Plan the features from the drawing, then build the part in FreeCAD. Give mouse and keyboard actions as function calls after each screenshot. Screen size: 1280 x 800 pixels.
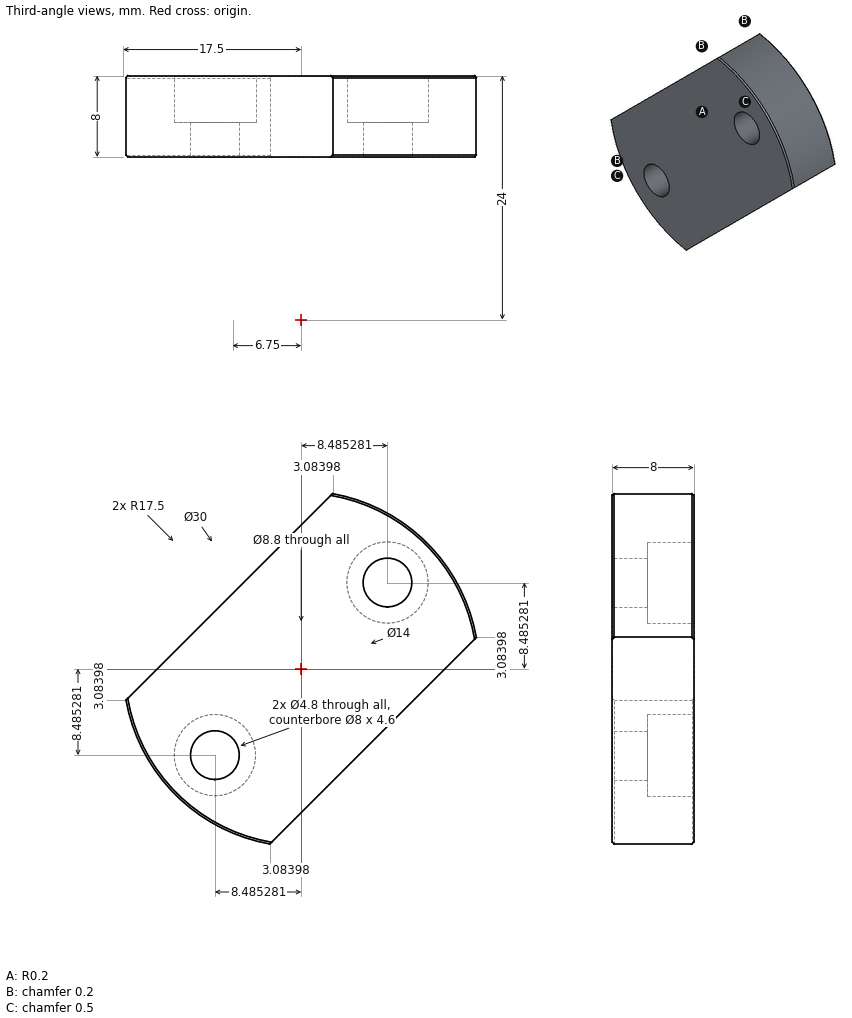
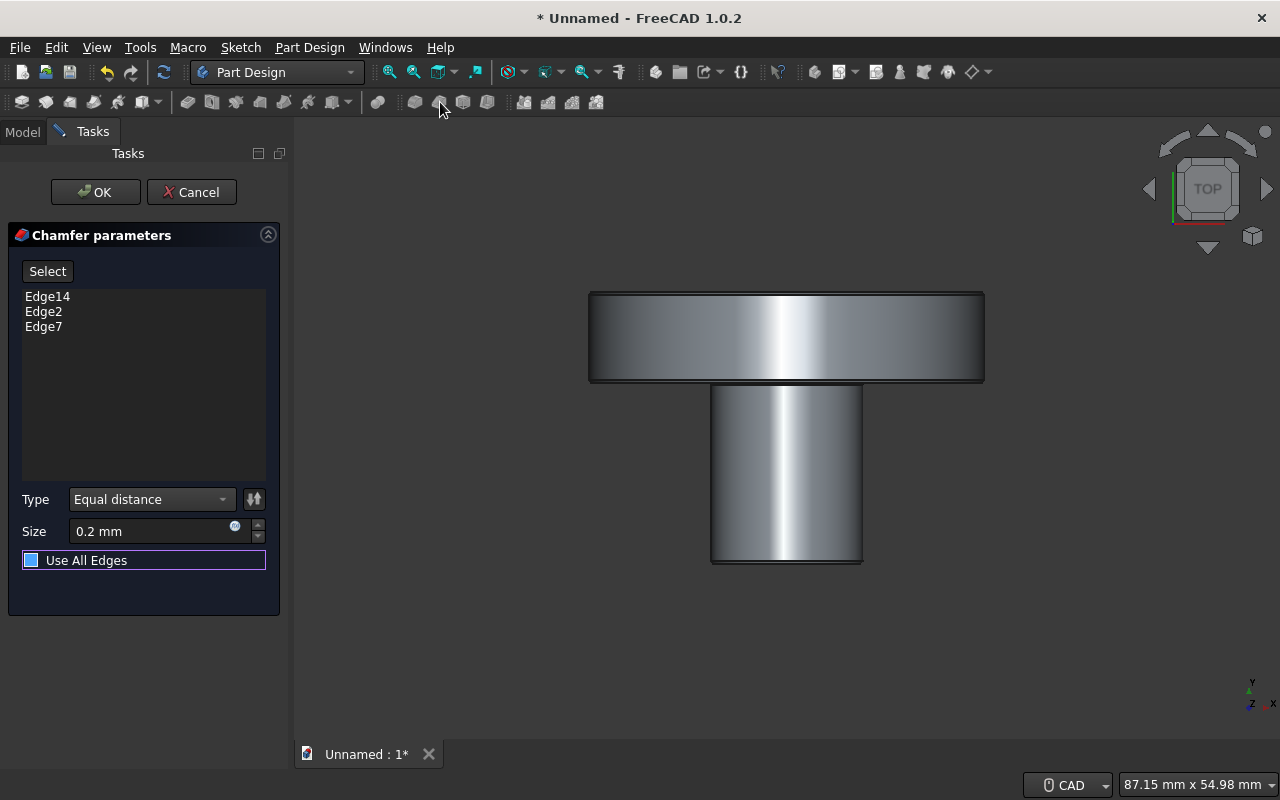
click(96, 192)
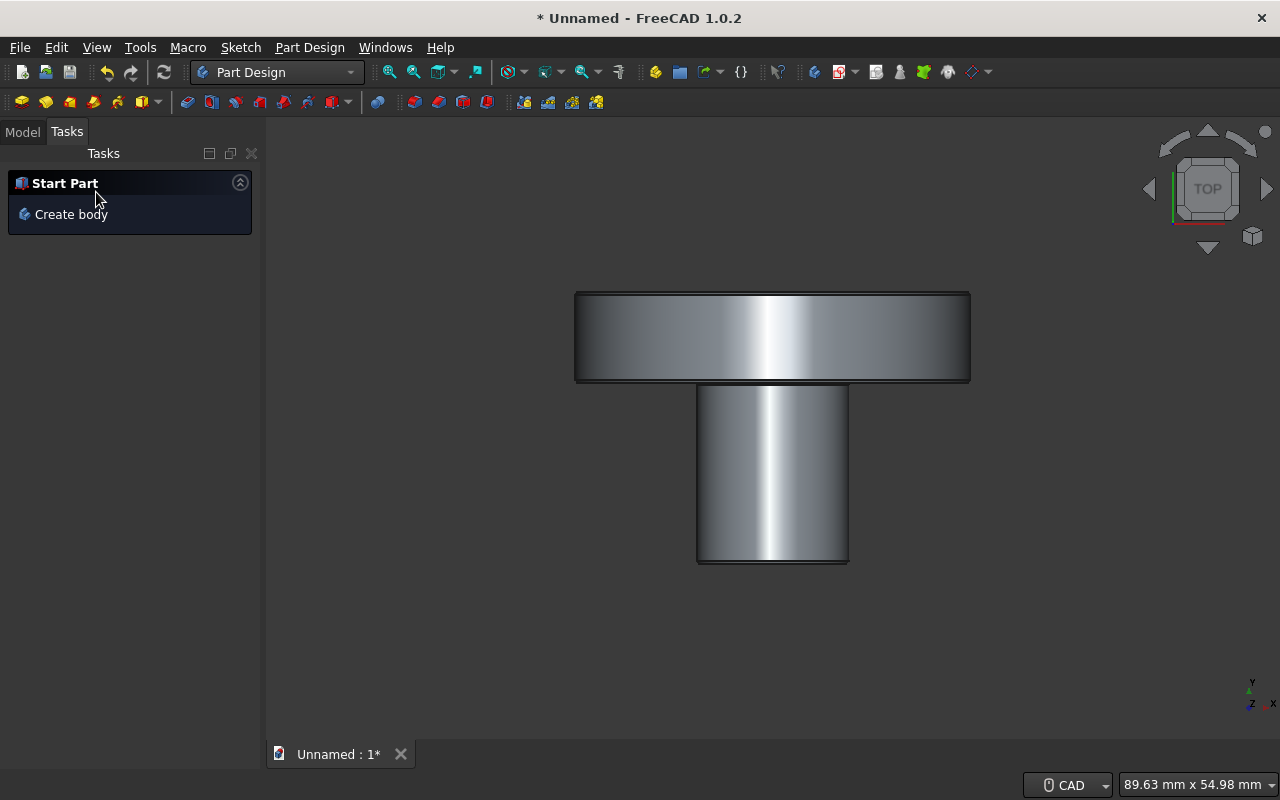
click(390, 72)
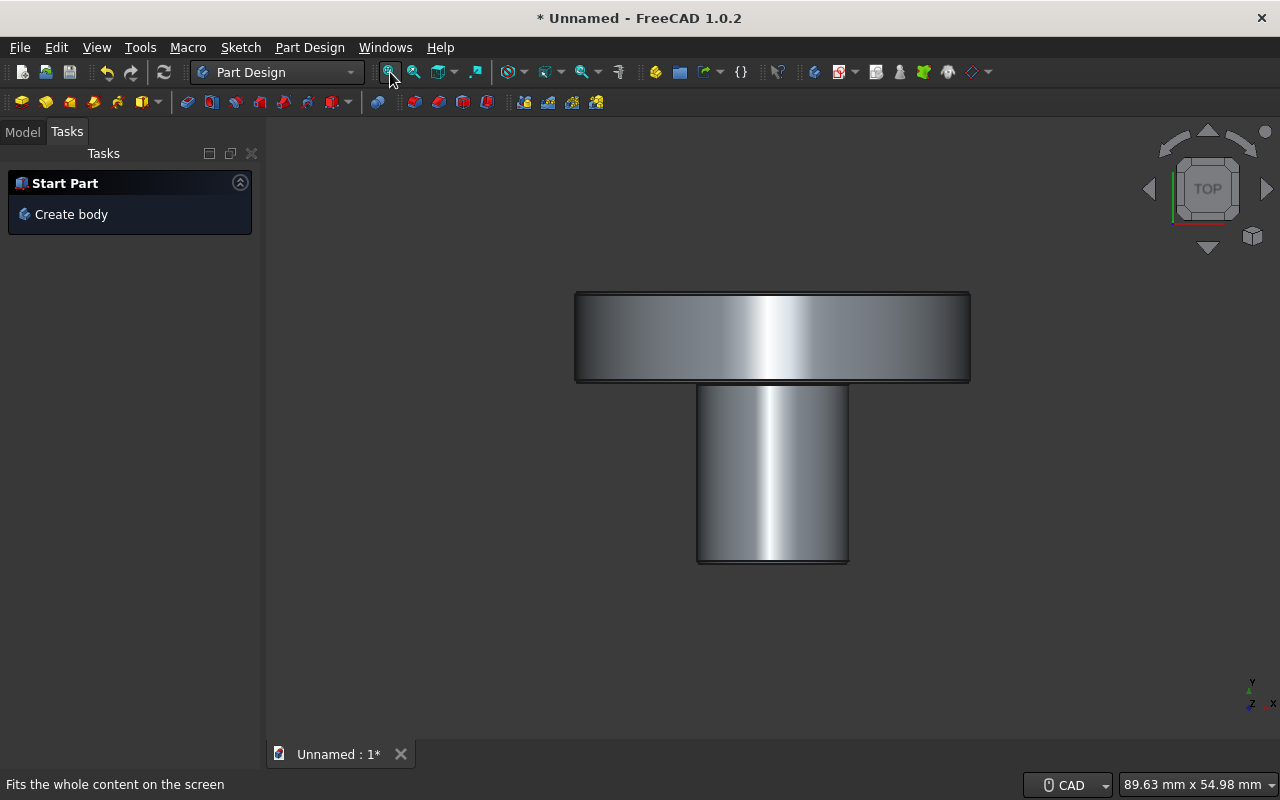
key(0)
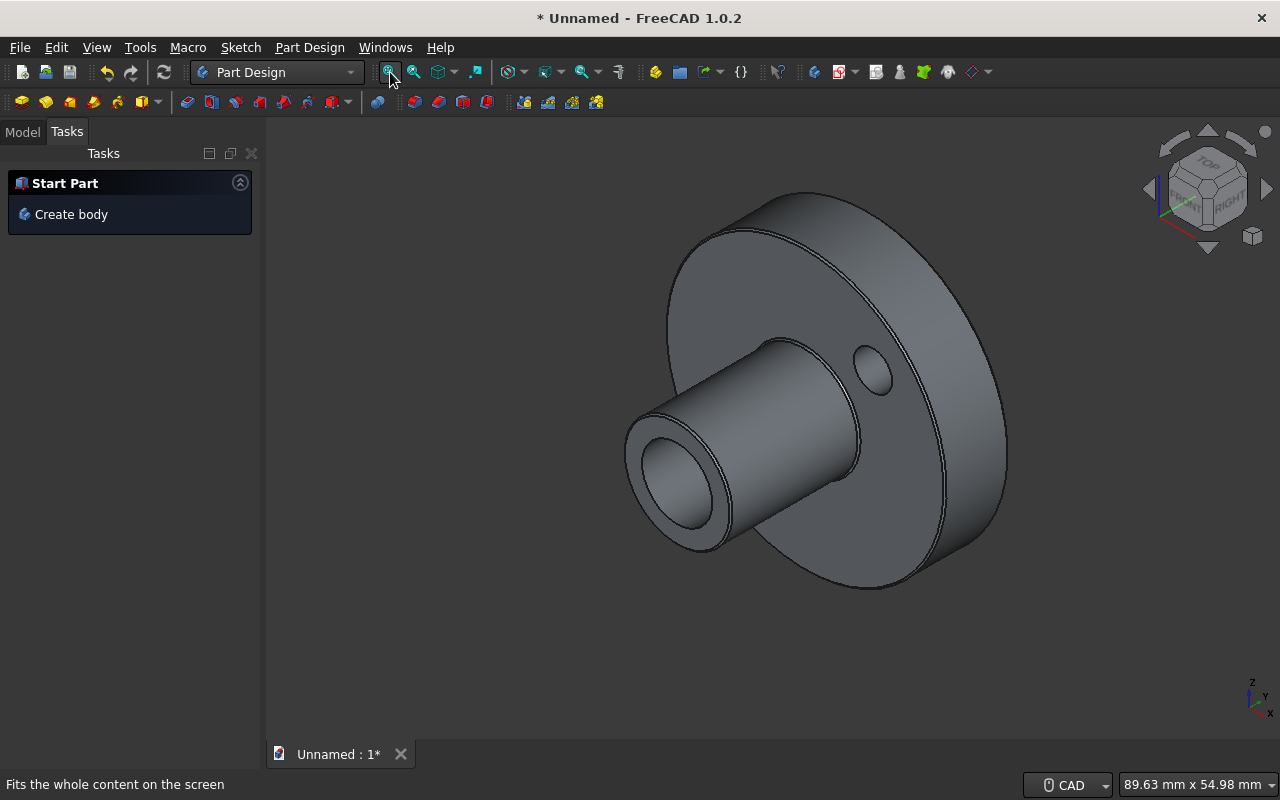
click(642, 462)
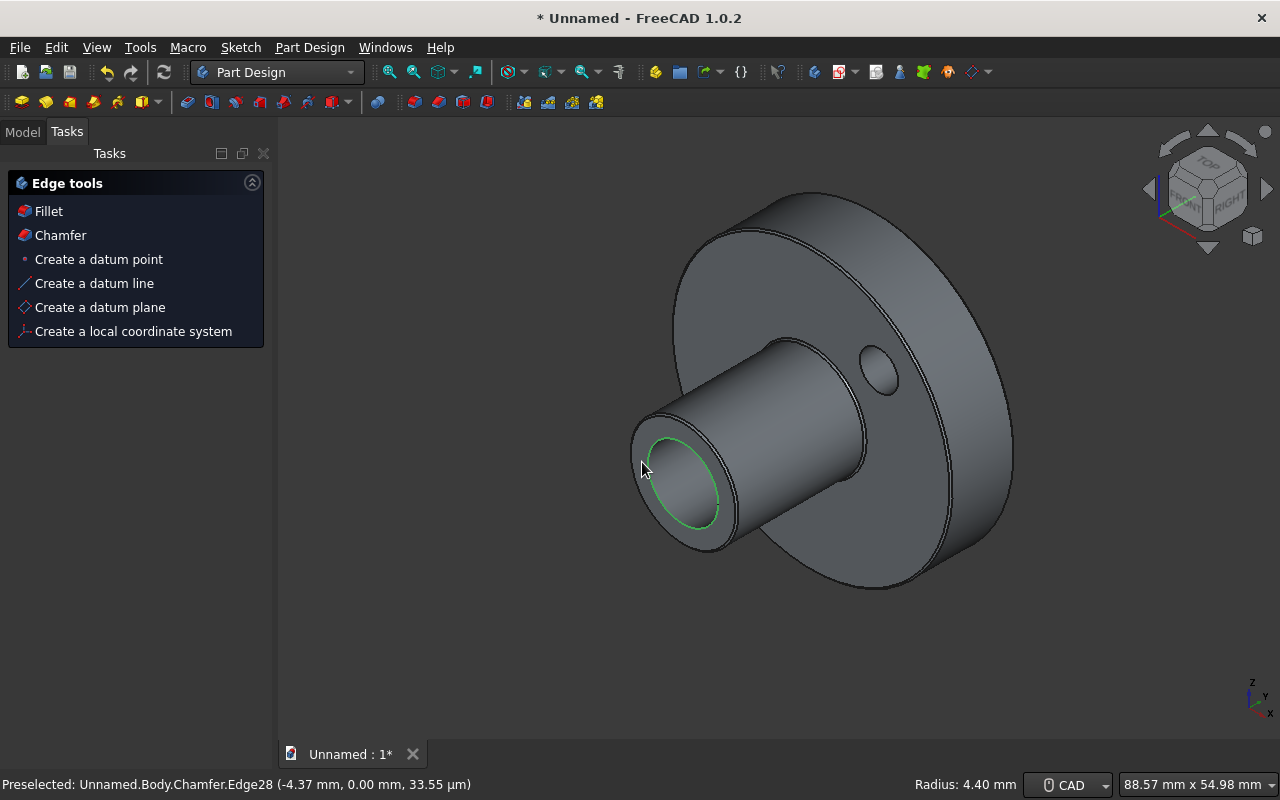
key(2)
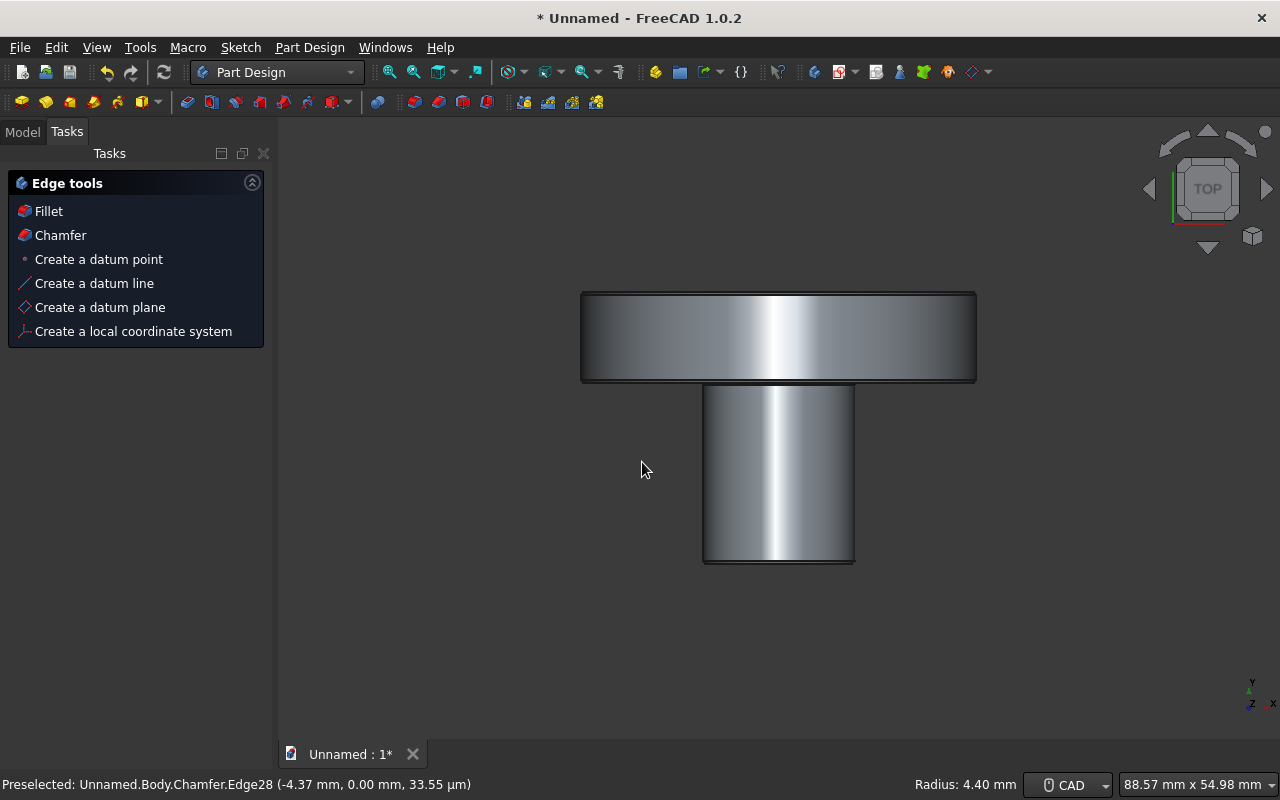
click(390, 72)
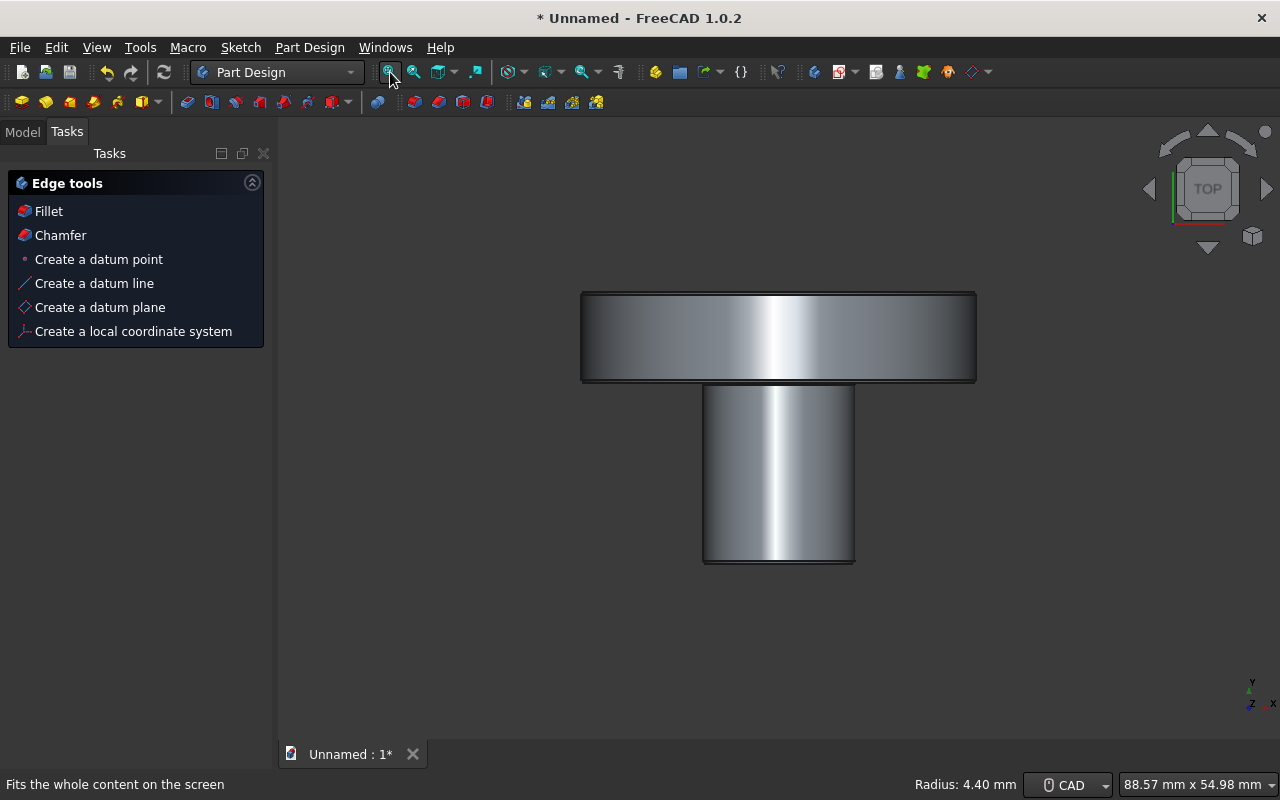
key(1)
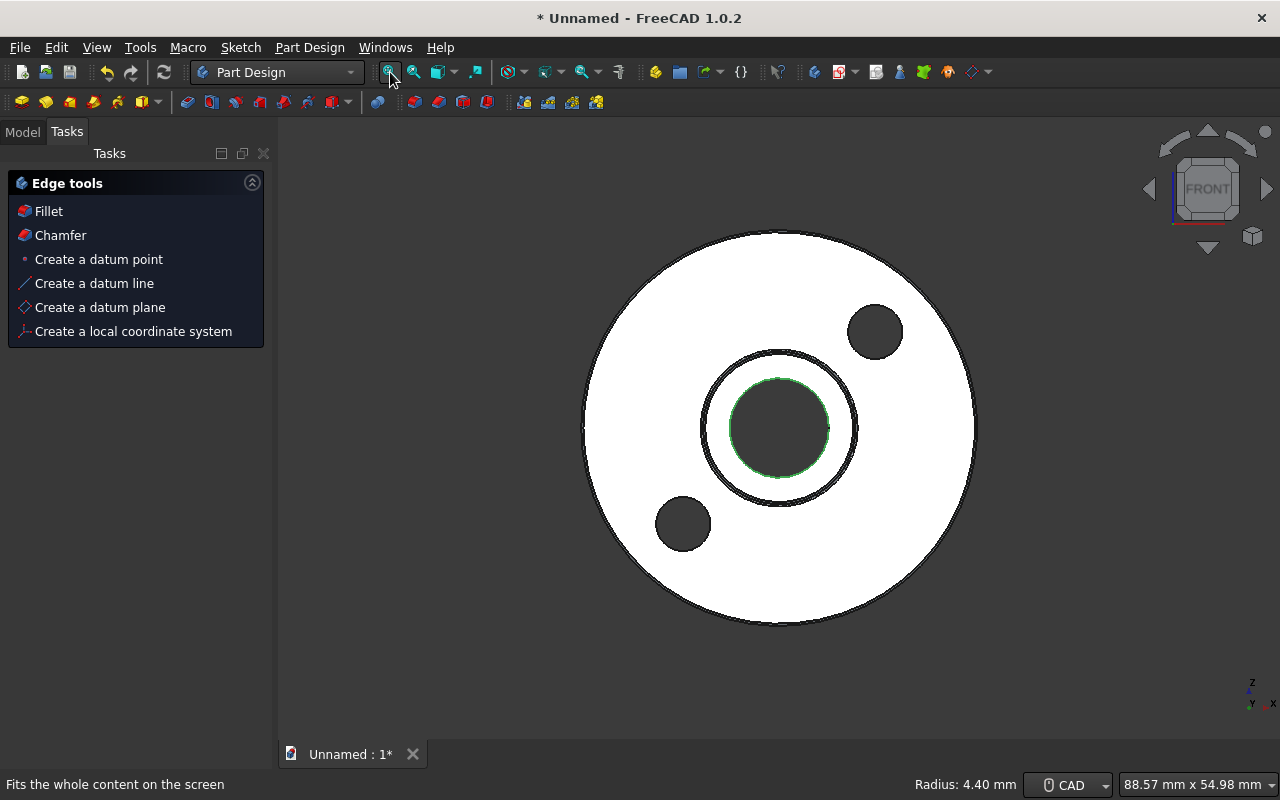
key(3)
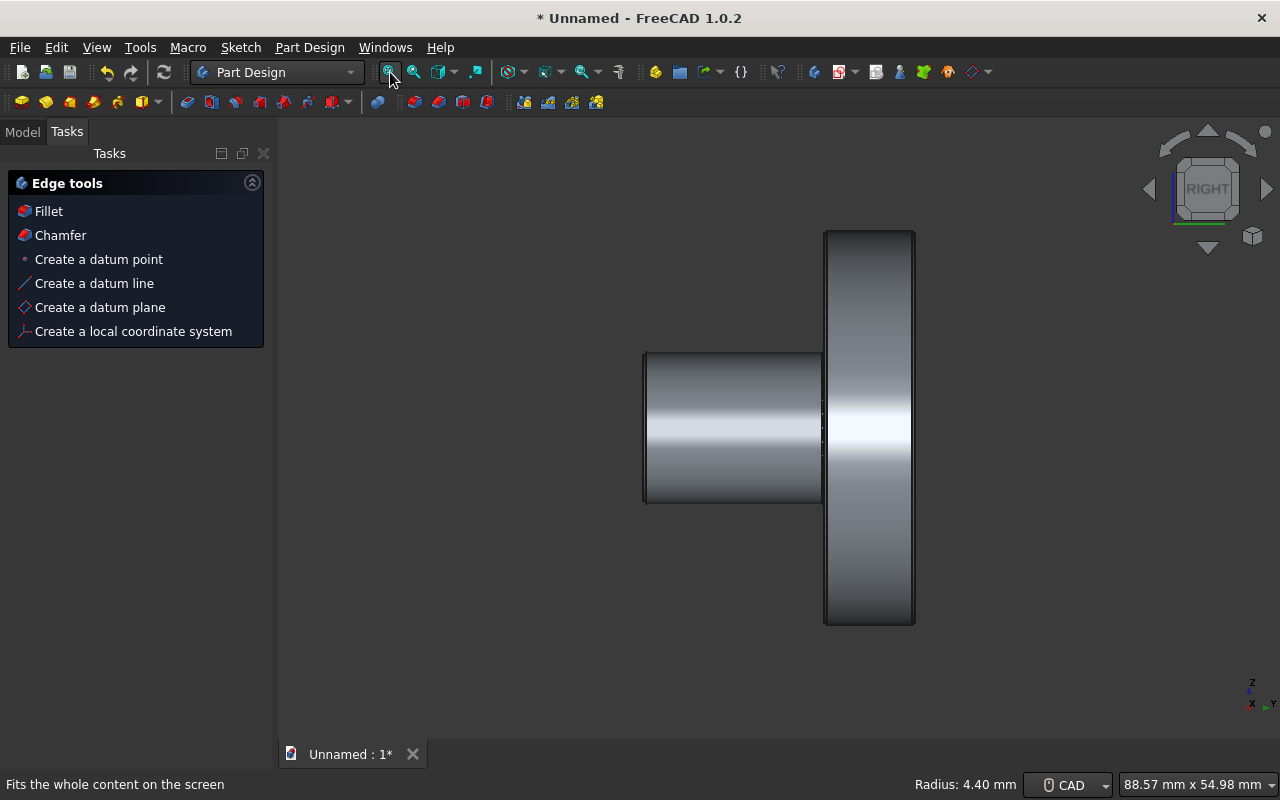
key(5)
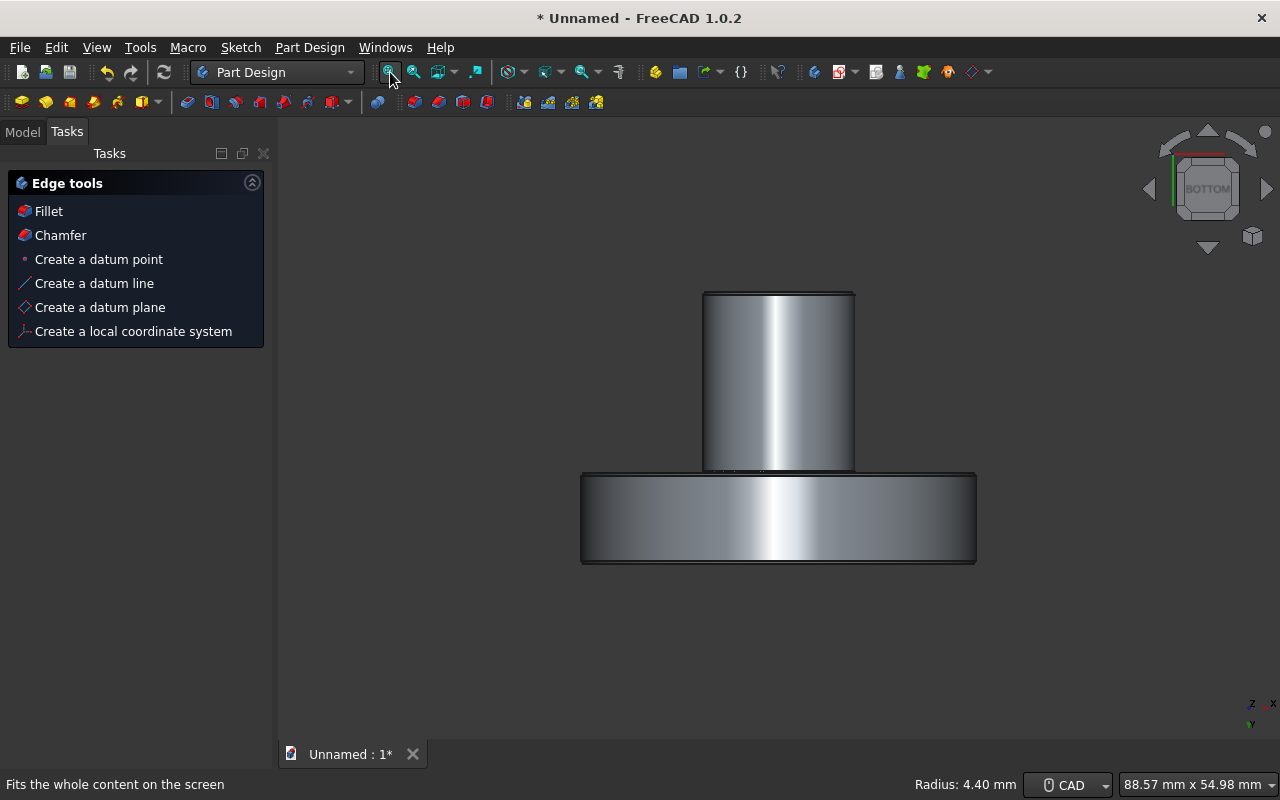
click(390, 72)